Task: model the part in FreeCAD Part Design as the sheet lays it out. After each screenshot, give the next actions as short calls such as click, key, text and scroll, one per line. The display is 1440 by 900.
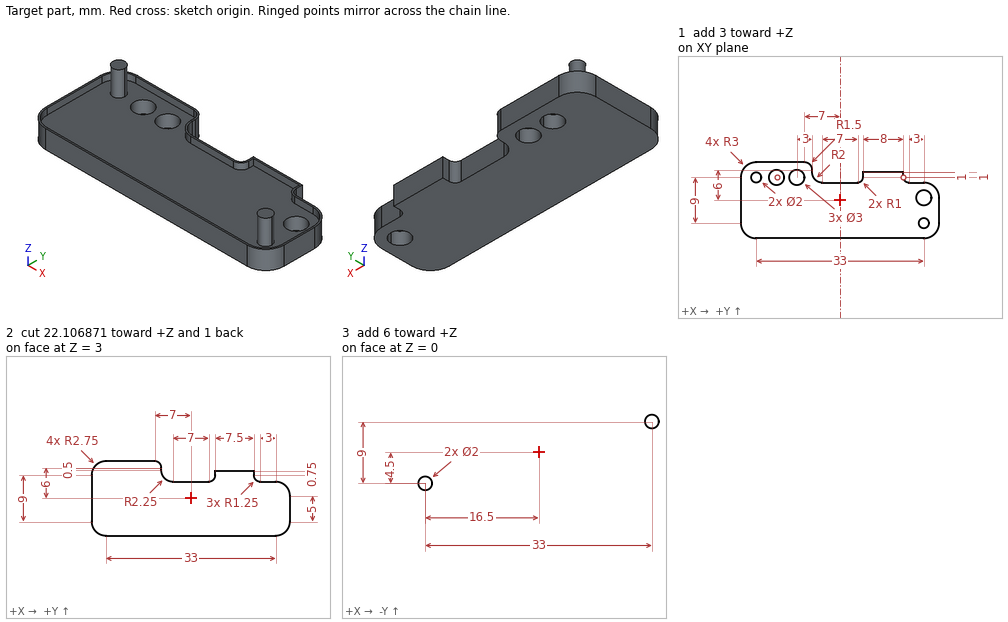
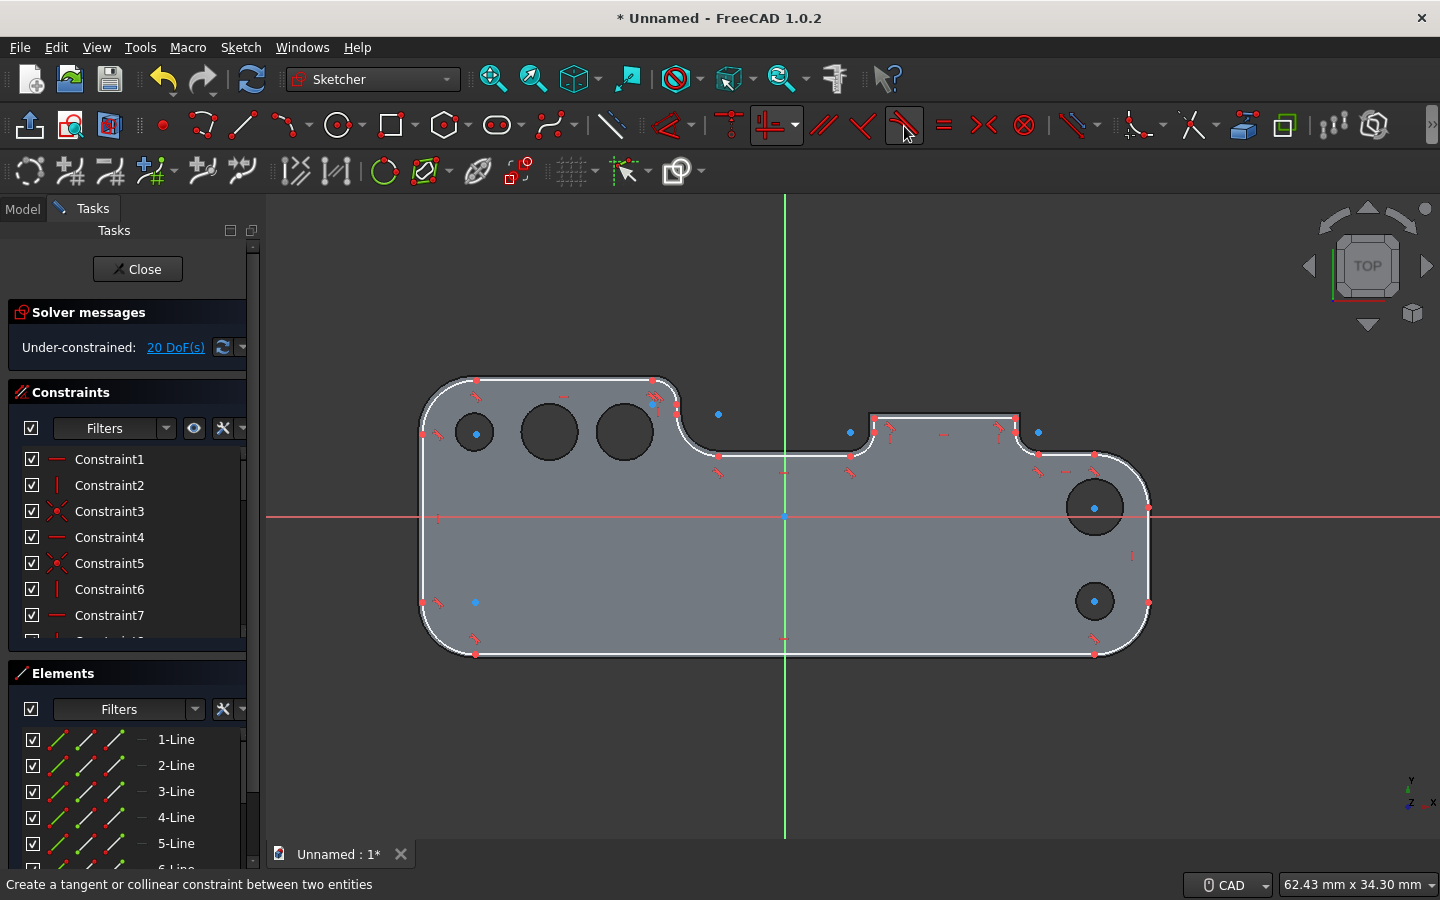
click(1148, 574)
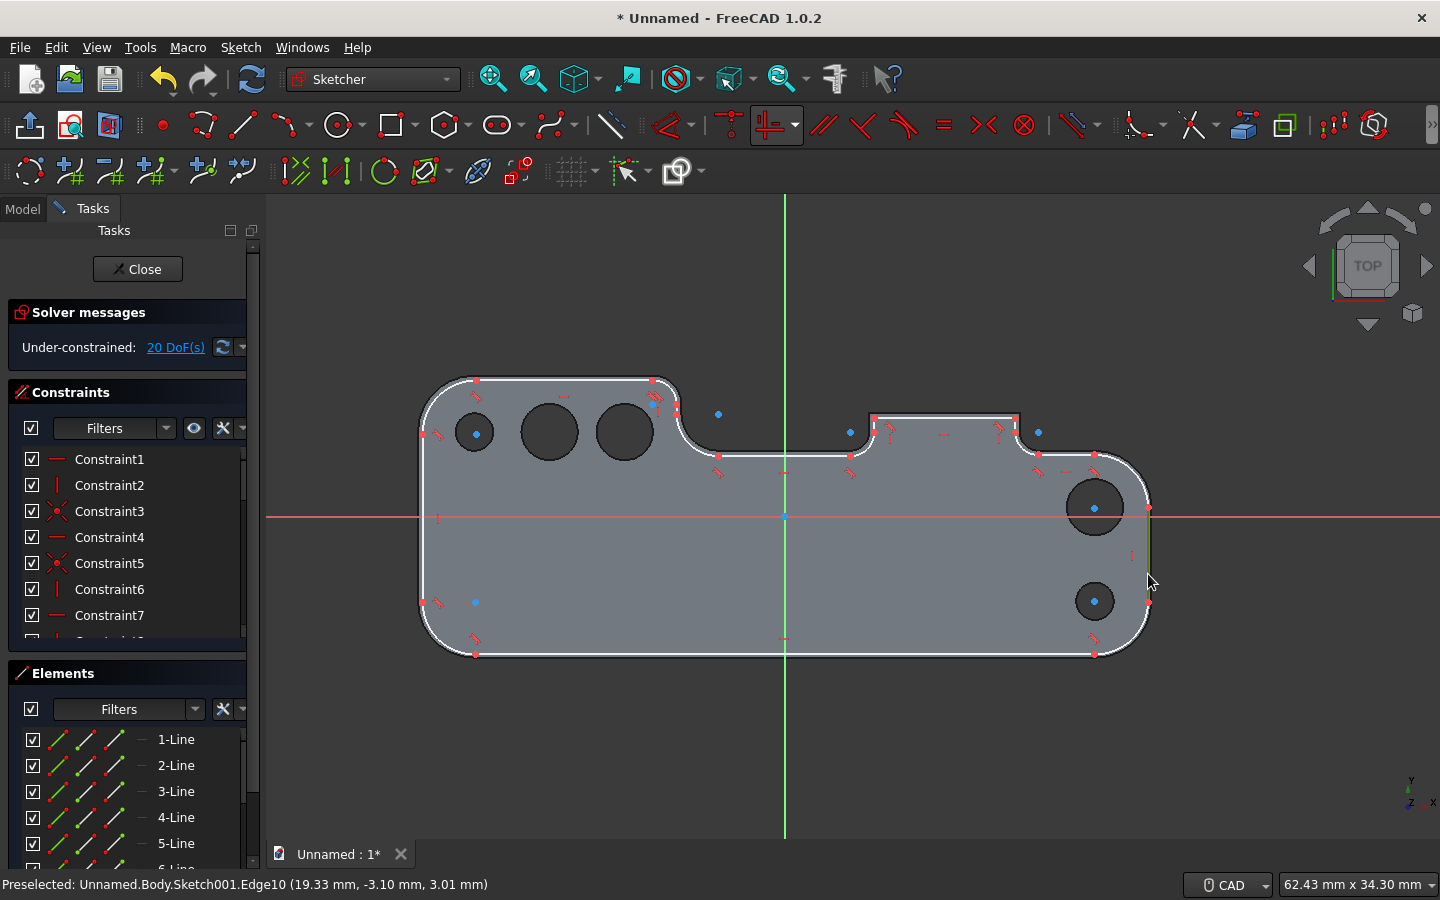
click(1119, 649)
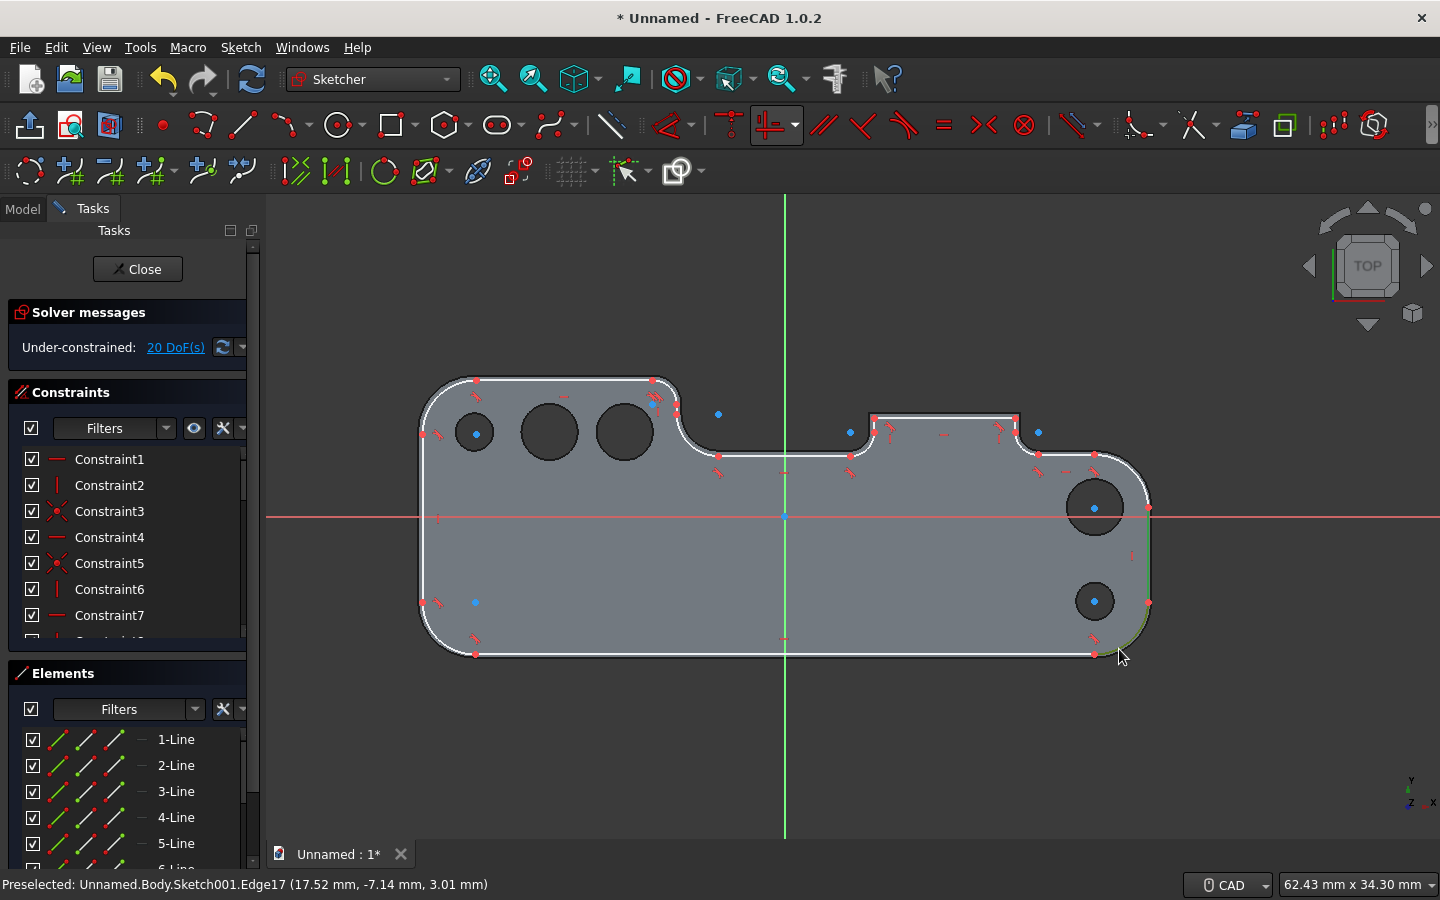
click(904, 126)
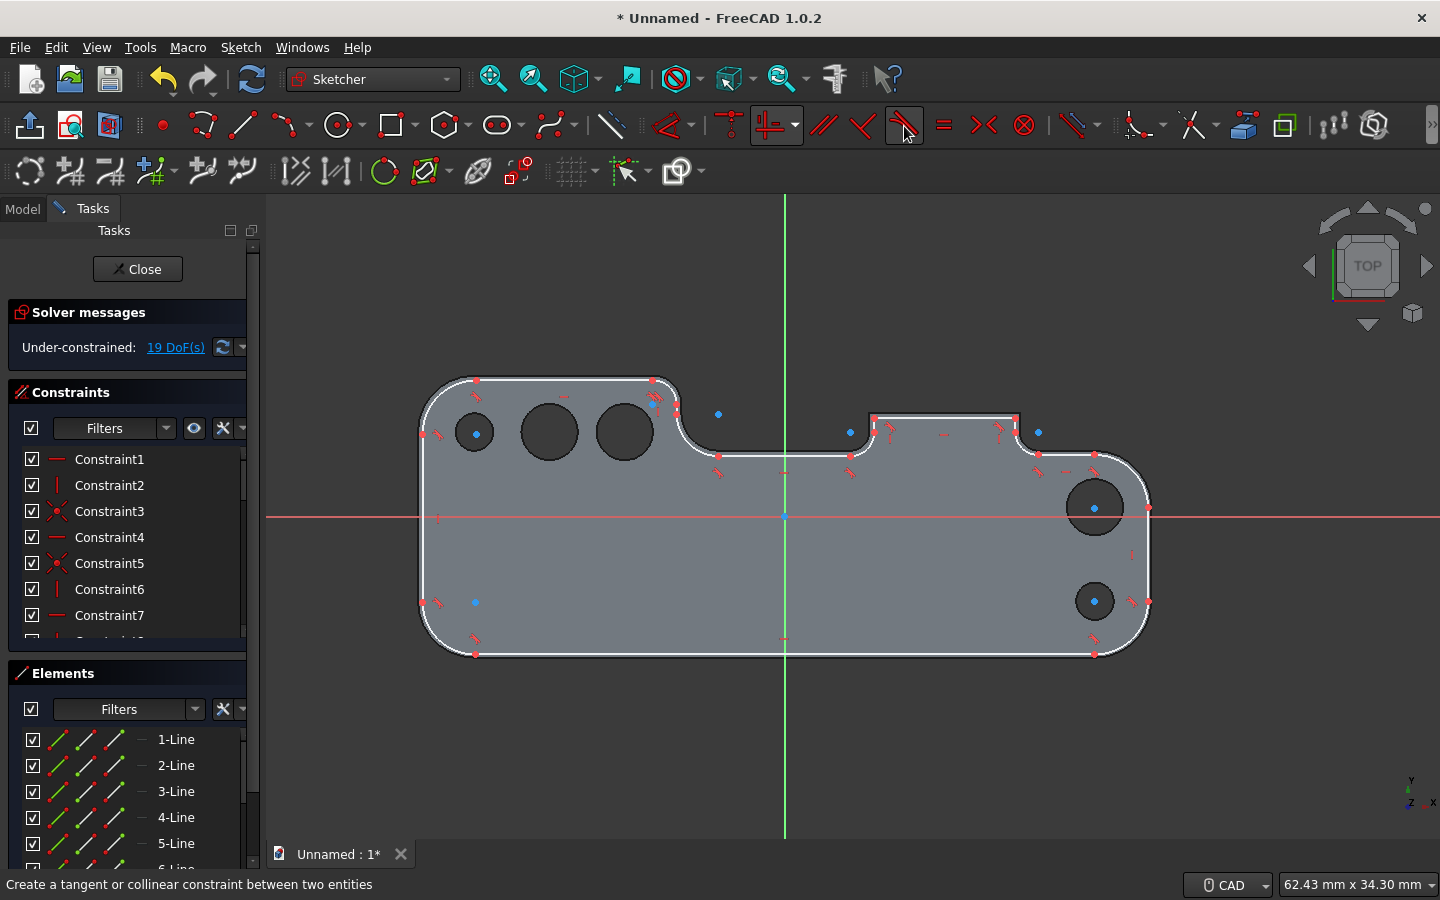
click(1148, 573)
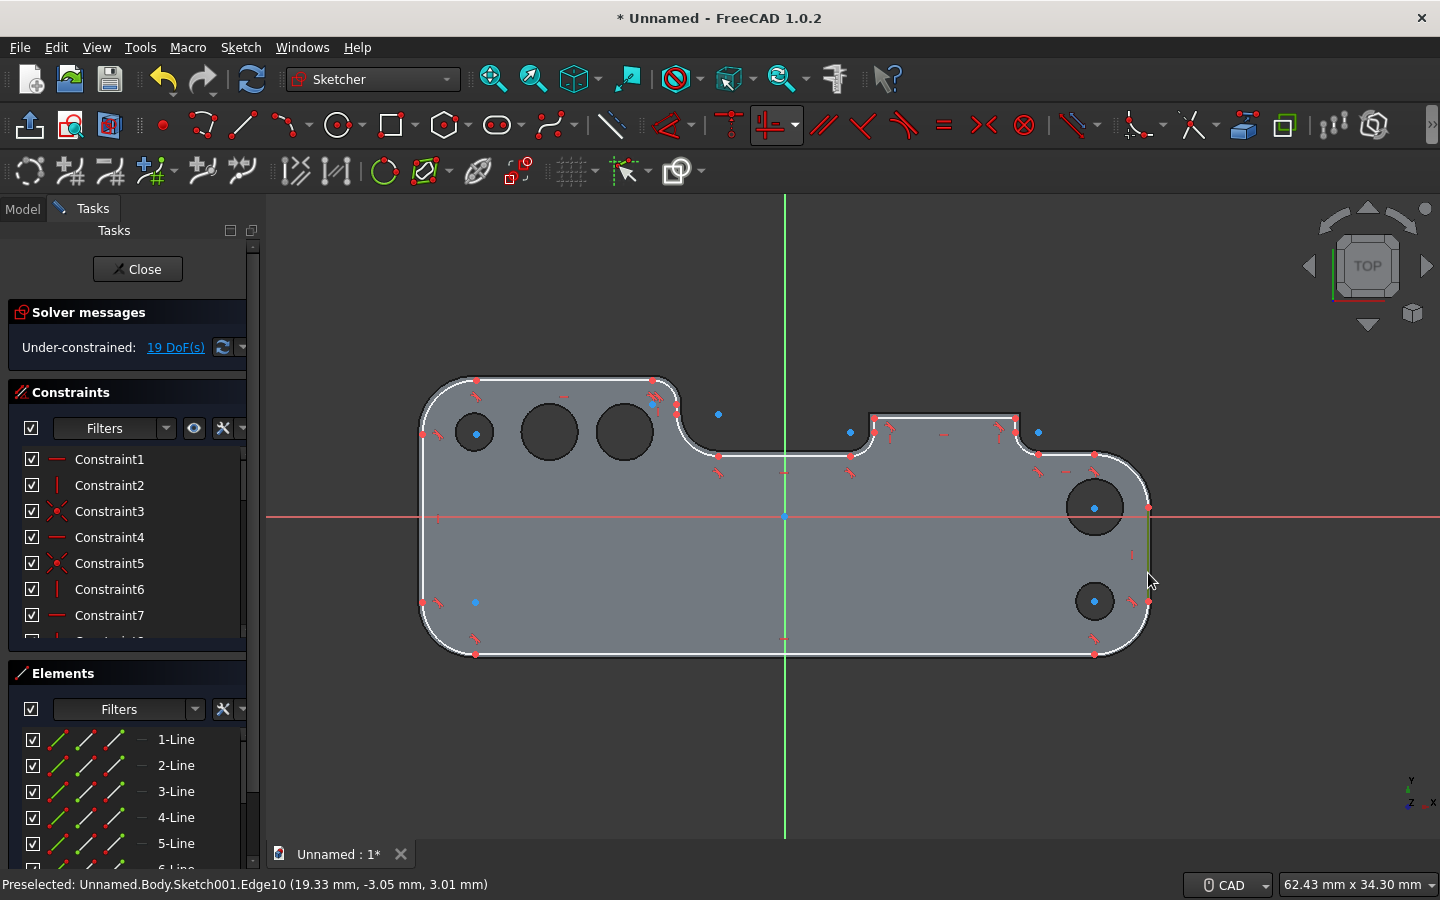
click(1142, 484)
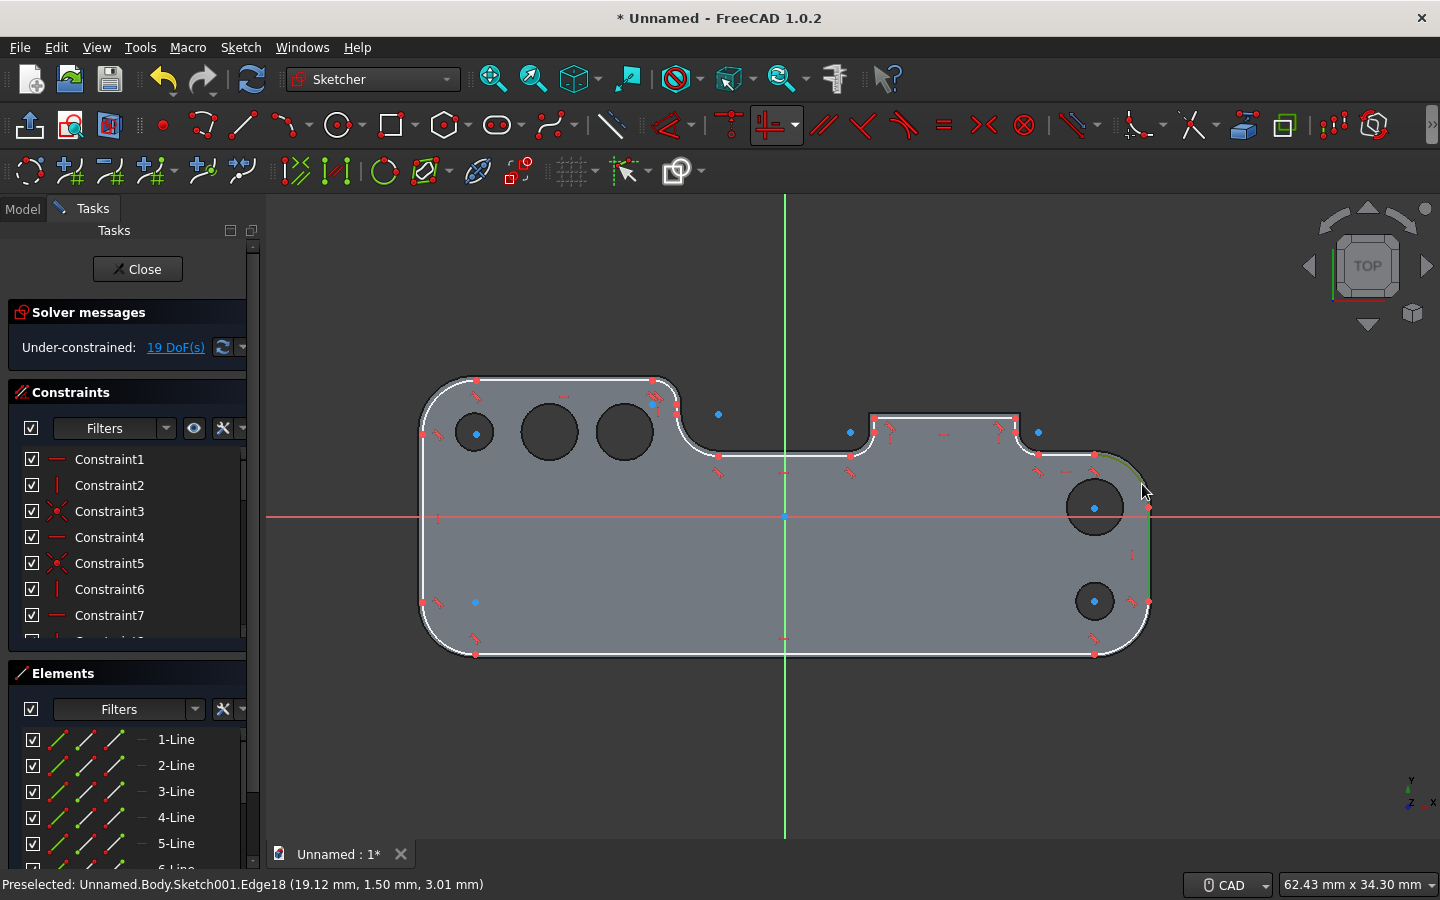
key(t)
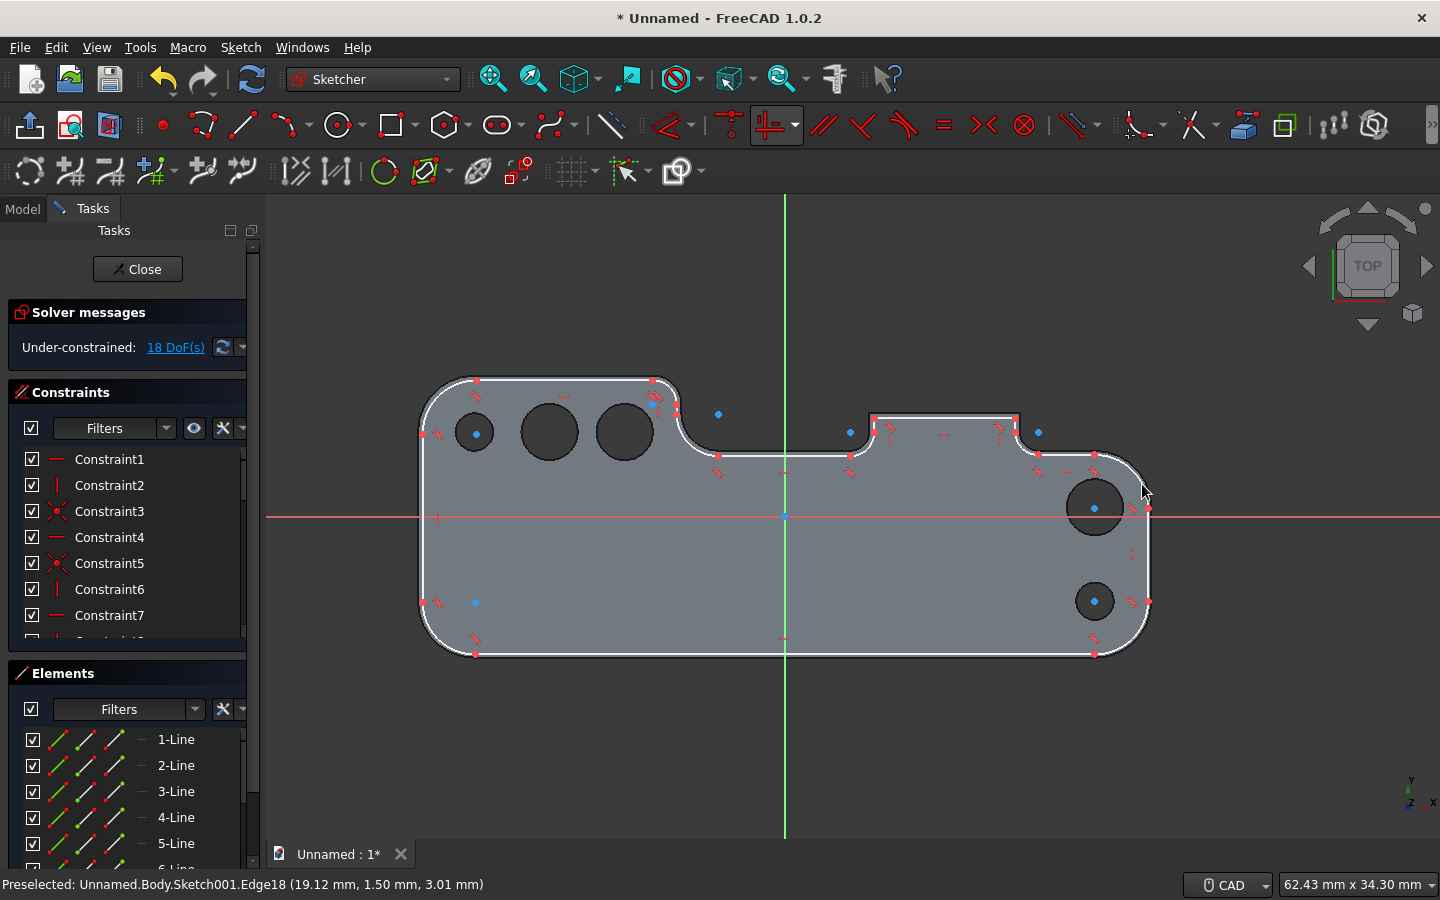
scroll(1018, 442, up, 2)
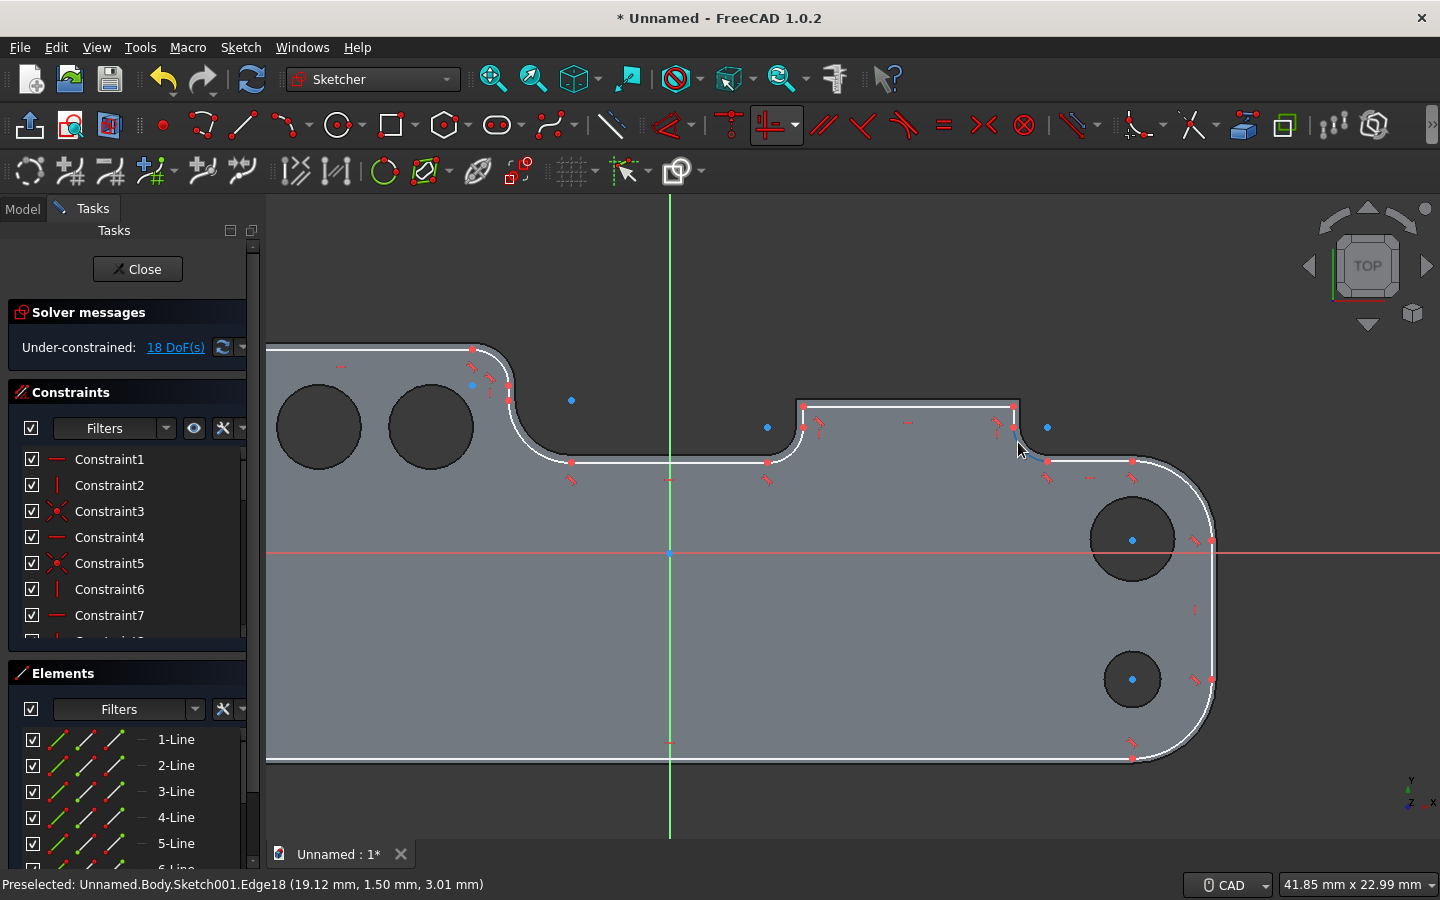
click(1018, 443)